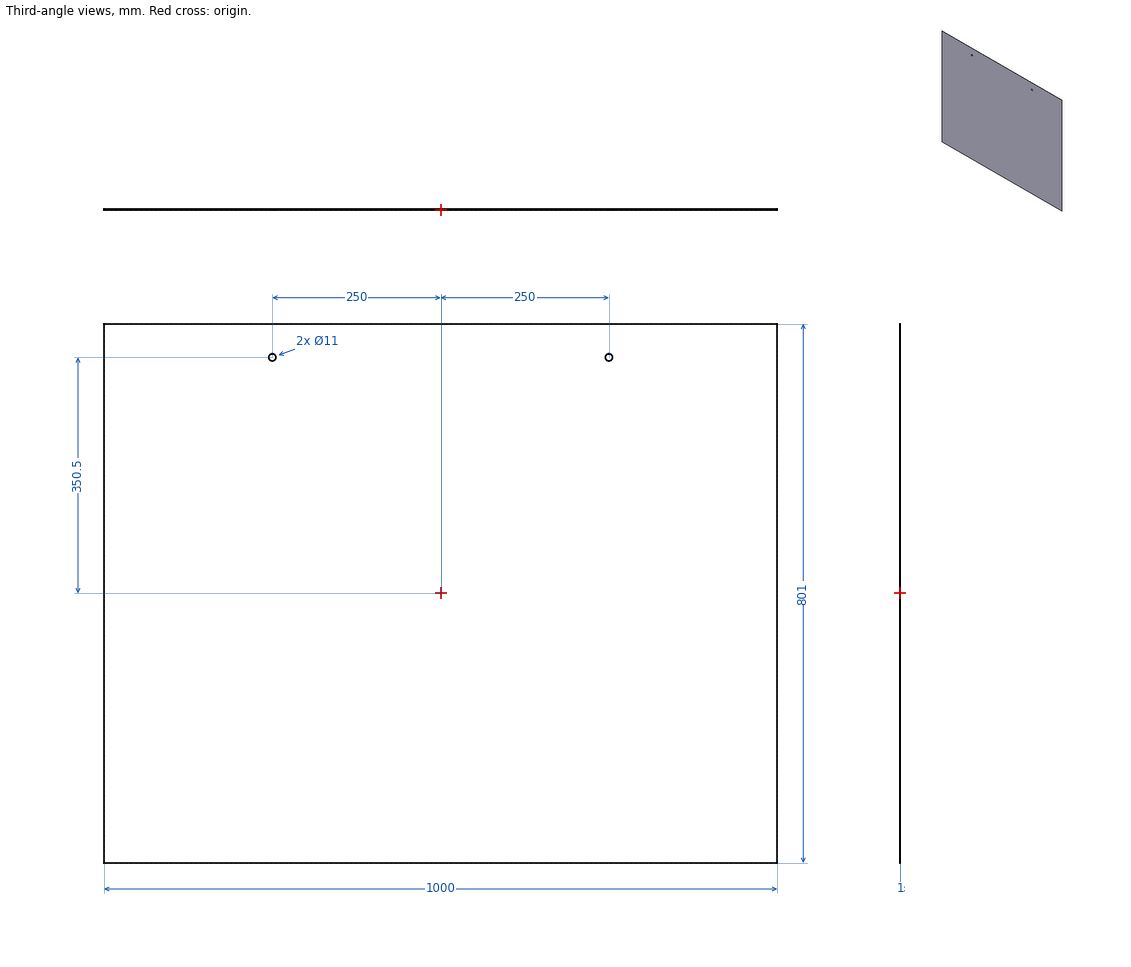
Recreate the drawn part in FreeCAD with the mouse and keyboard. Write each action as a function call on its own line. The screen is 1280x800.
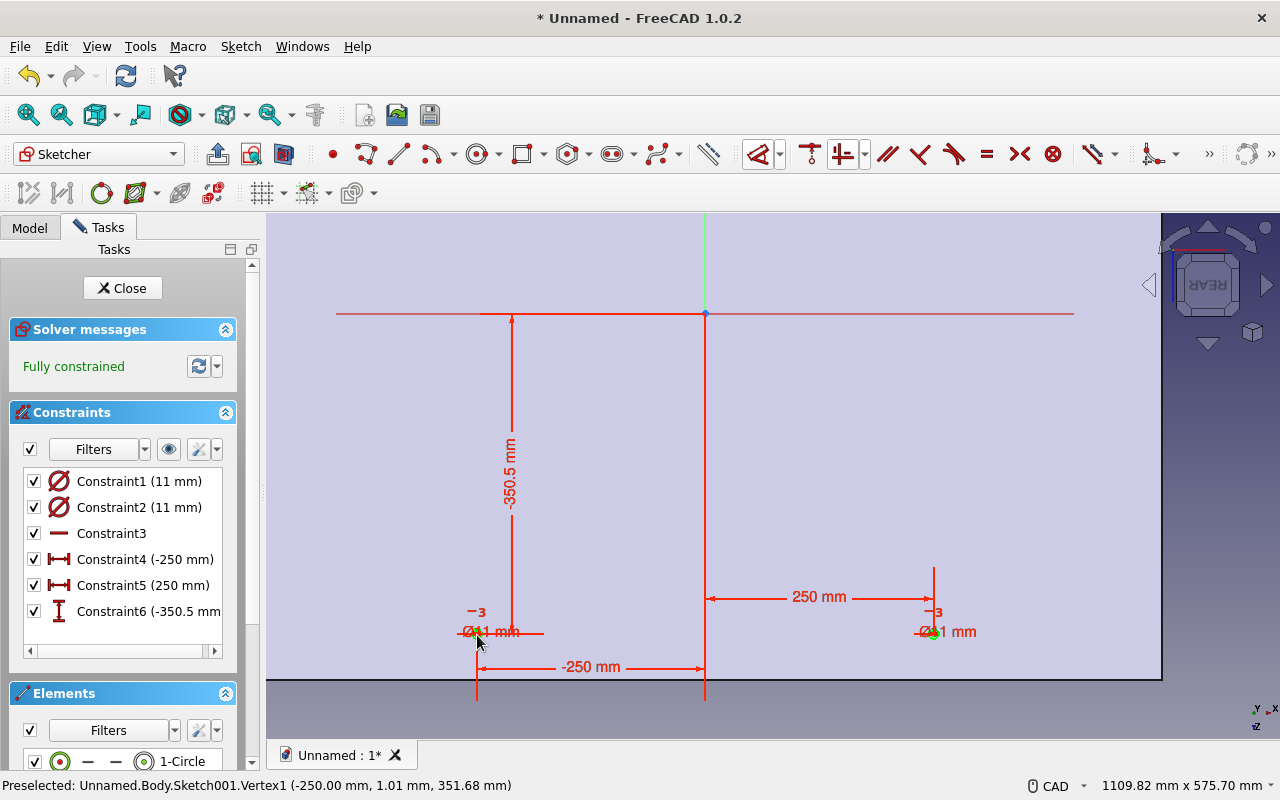
click(123, 288)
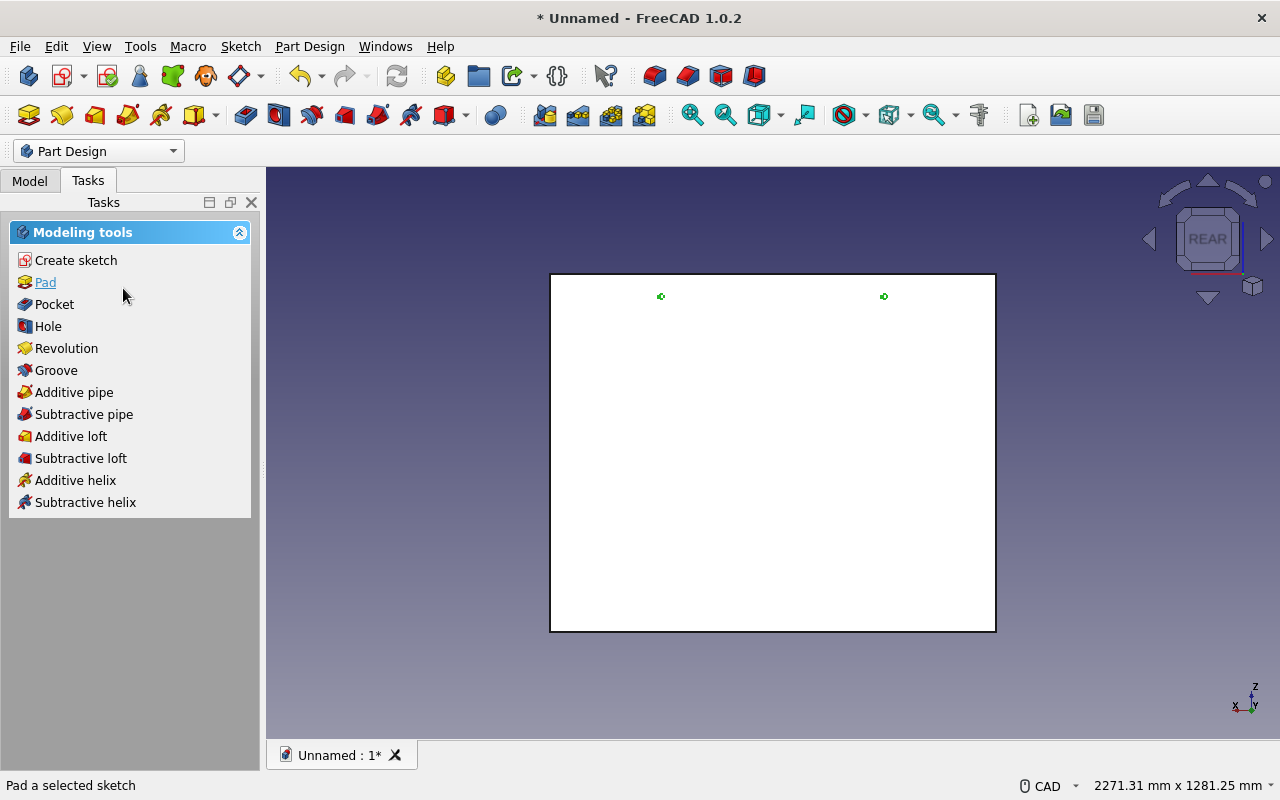
click(246, 116)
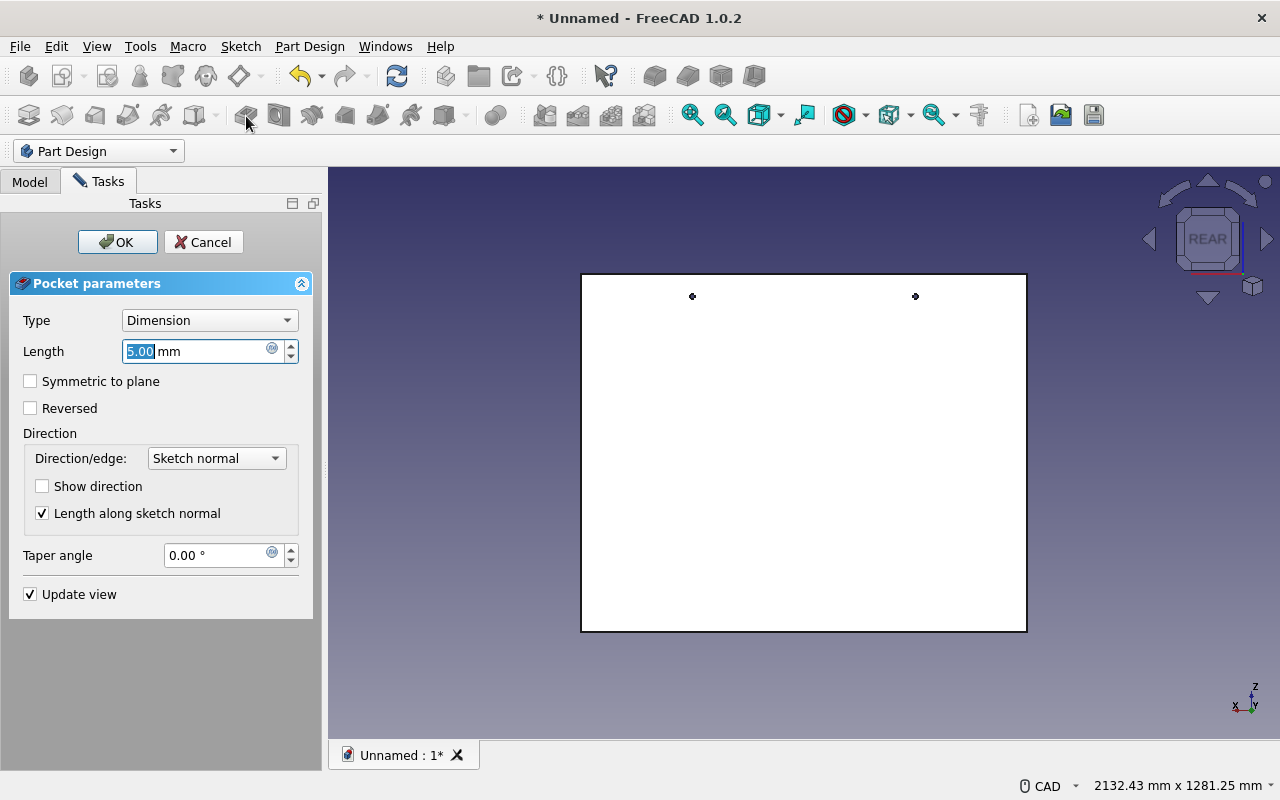
click(210, 320)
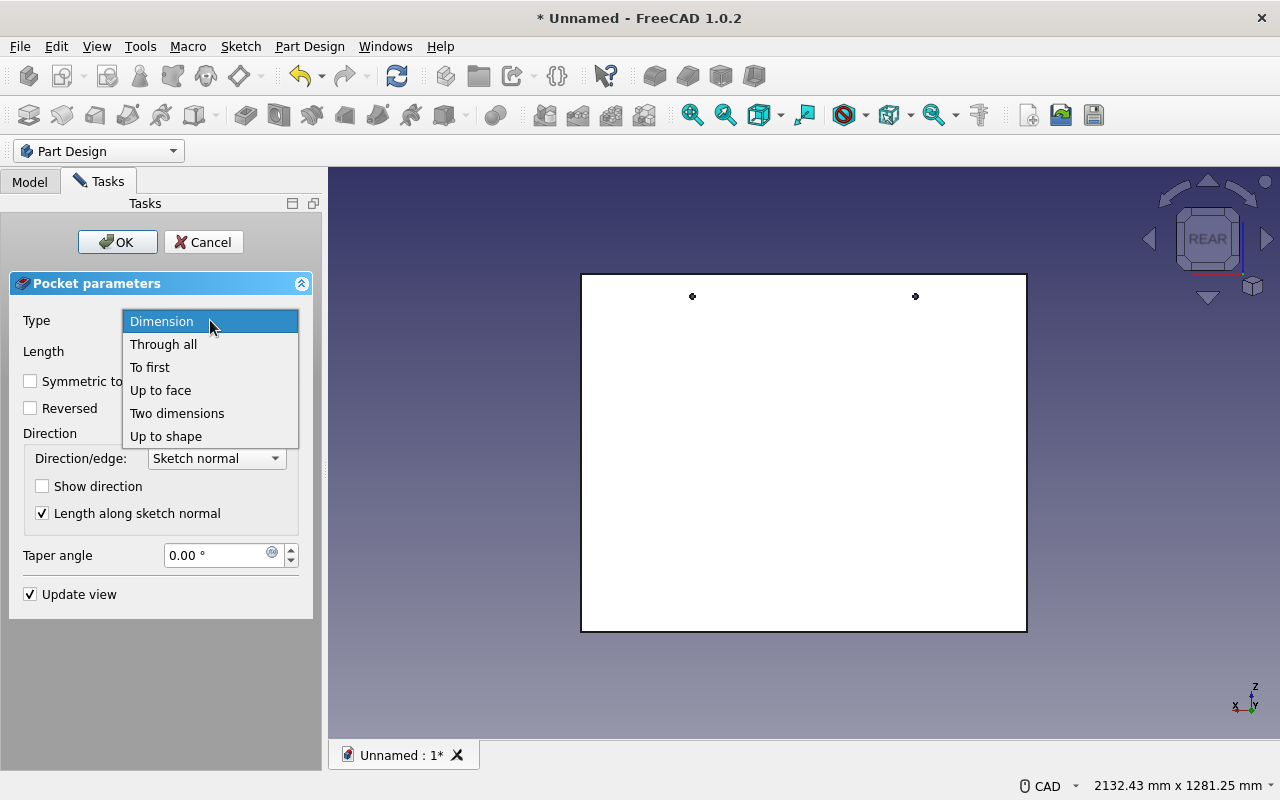
click(208, 344)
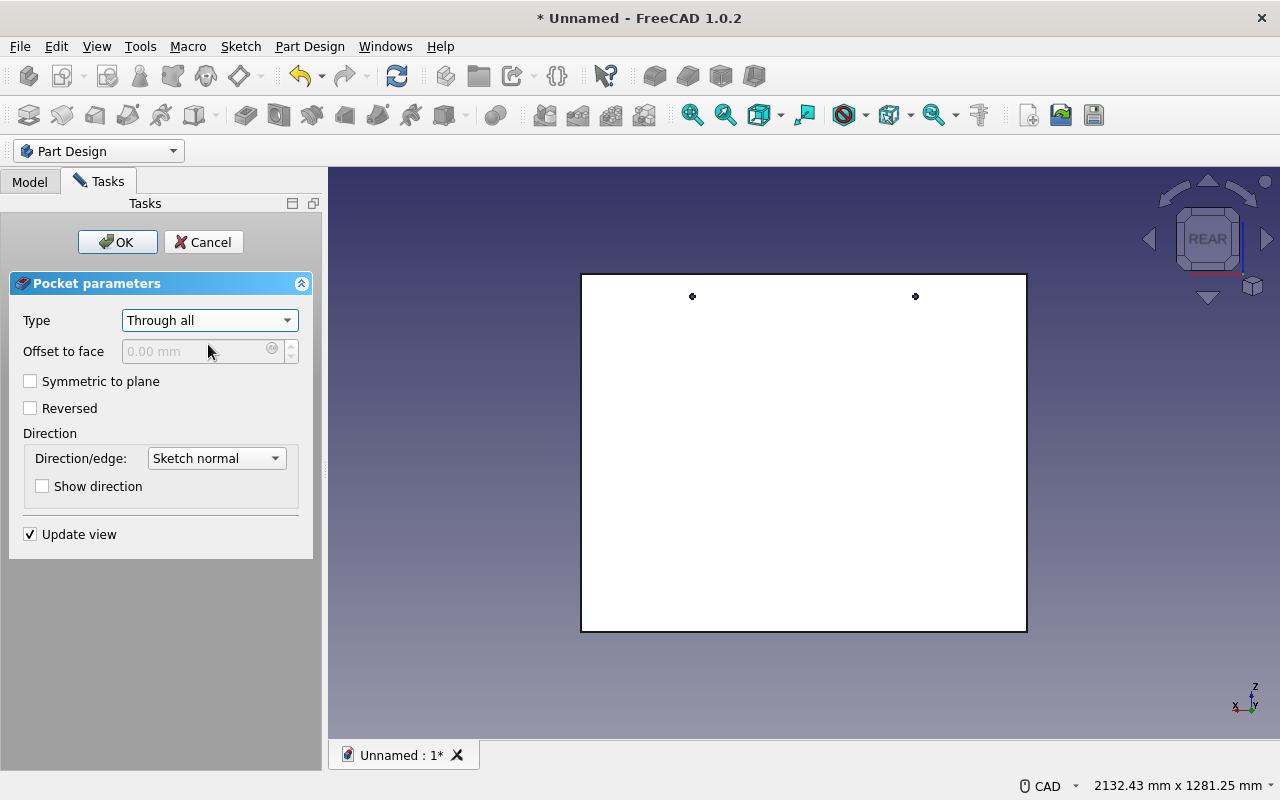
click(118, 242)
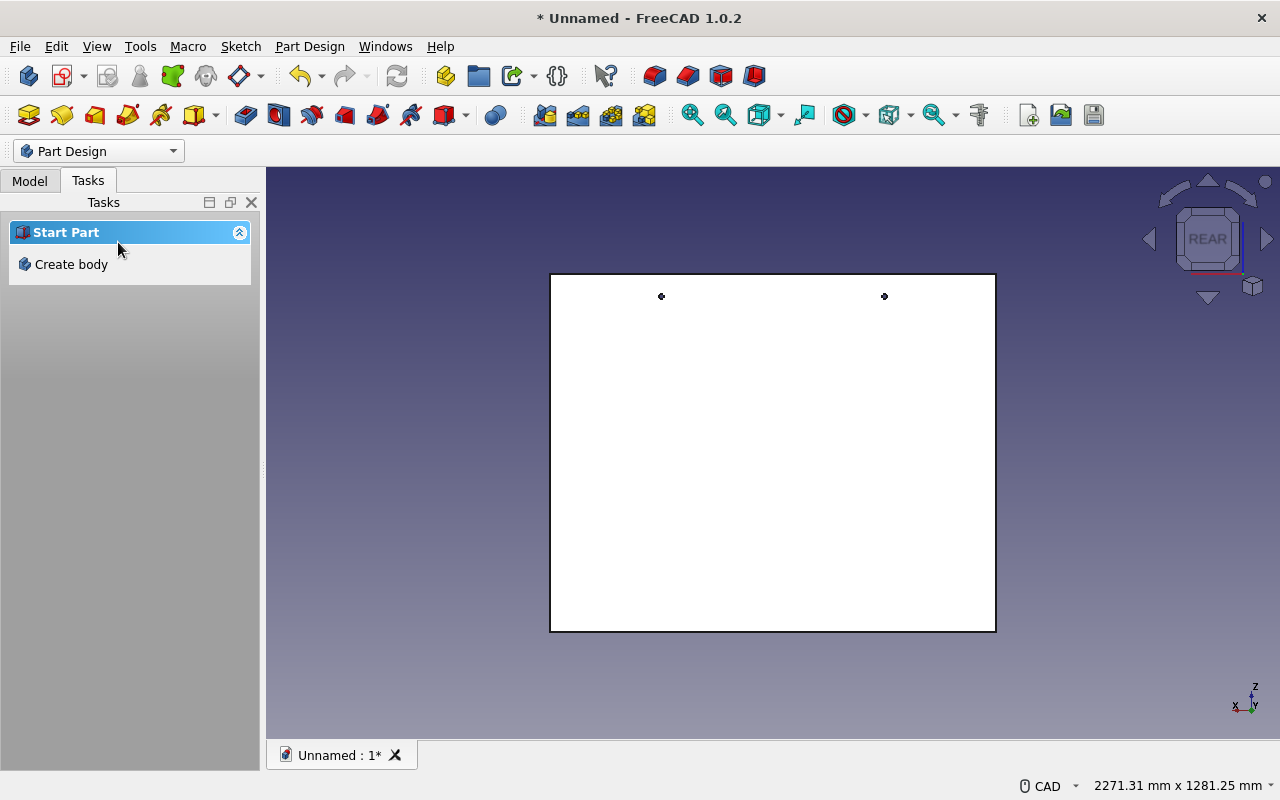
key(0)